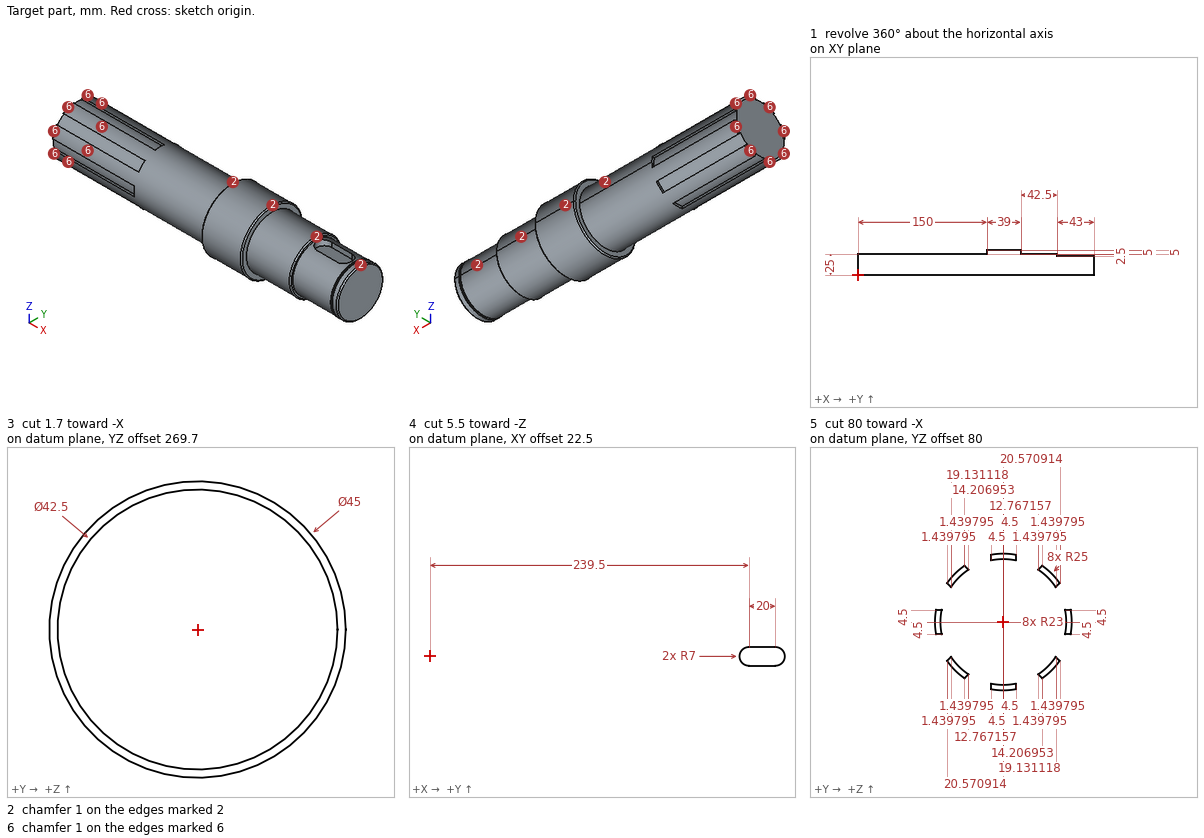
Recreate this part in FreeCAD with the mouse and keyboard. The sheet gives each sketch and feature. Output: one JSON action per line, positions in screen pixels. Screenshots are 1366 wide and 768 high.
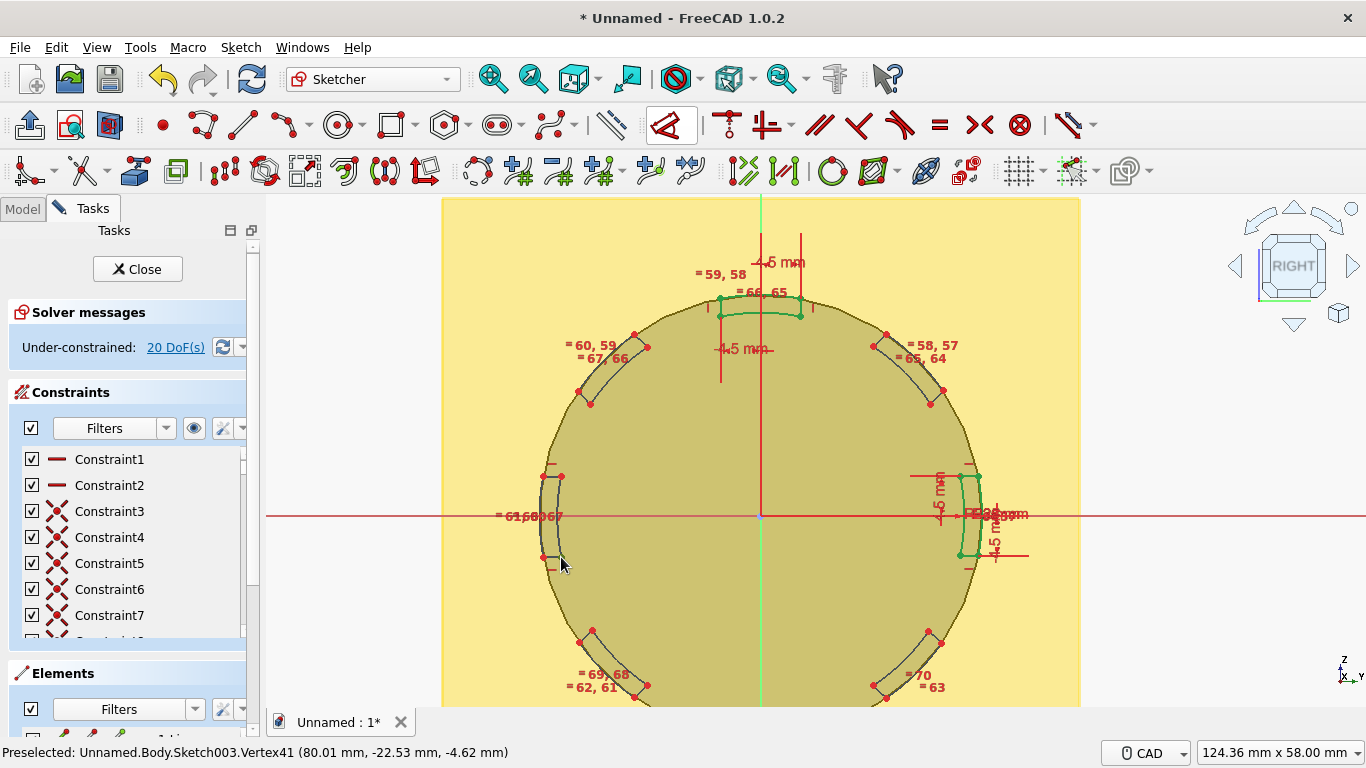
{"action": "left_click", "coordinate": [692, 126]}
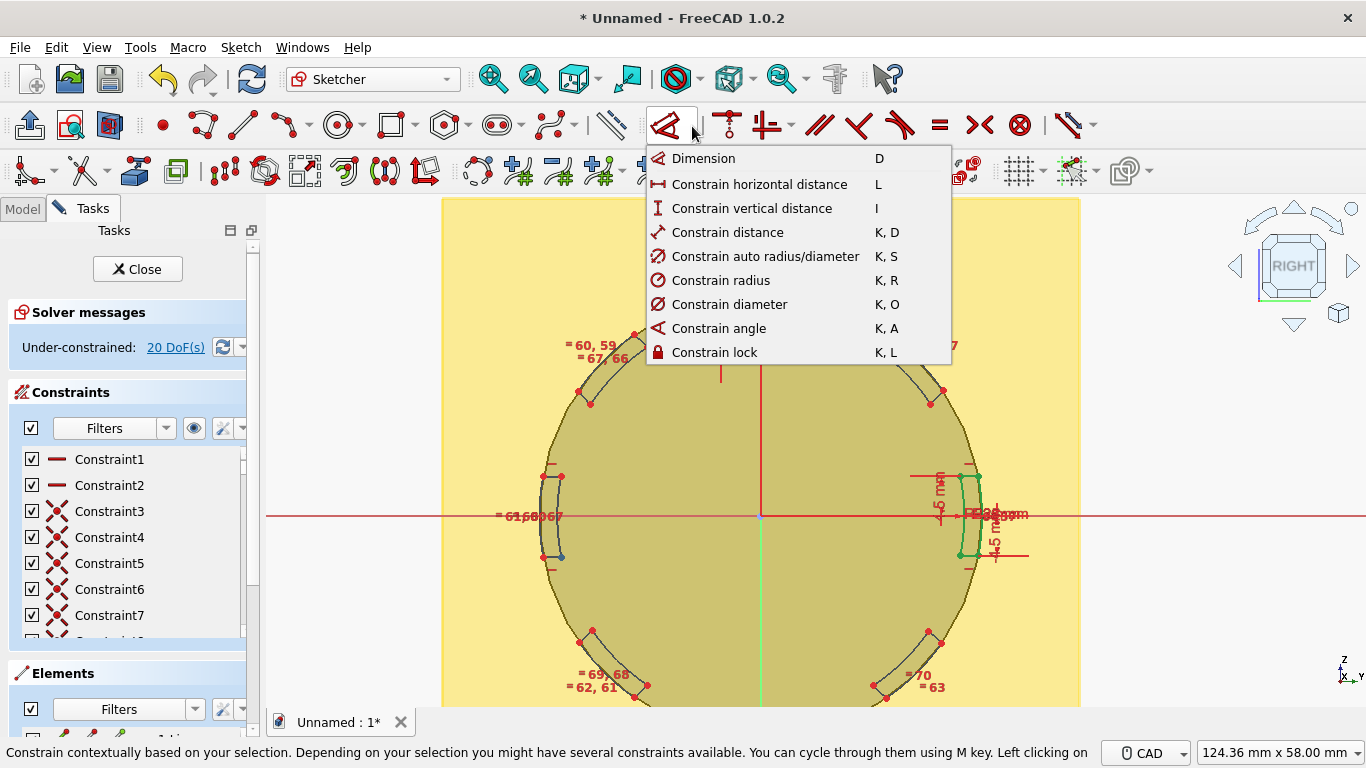
{"action": "left_click", "coordinate": [799, 208]}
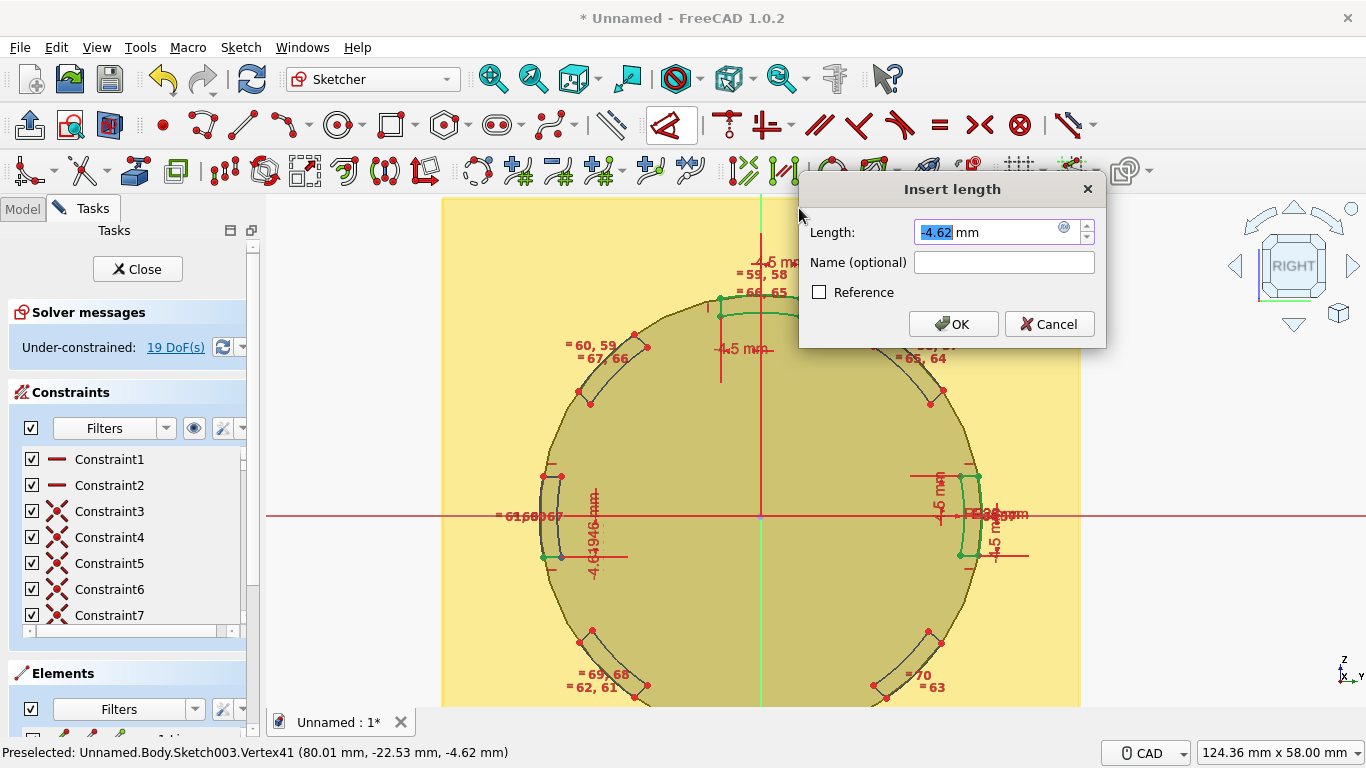
{"action": "type", "text": "-4.5"}
{"action": "key", "text": "Return"}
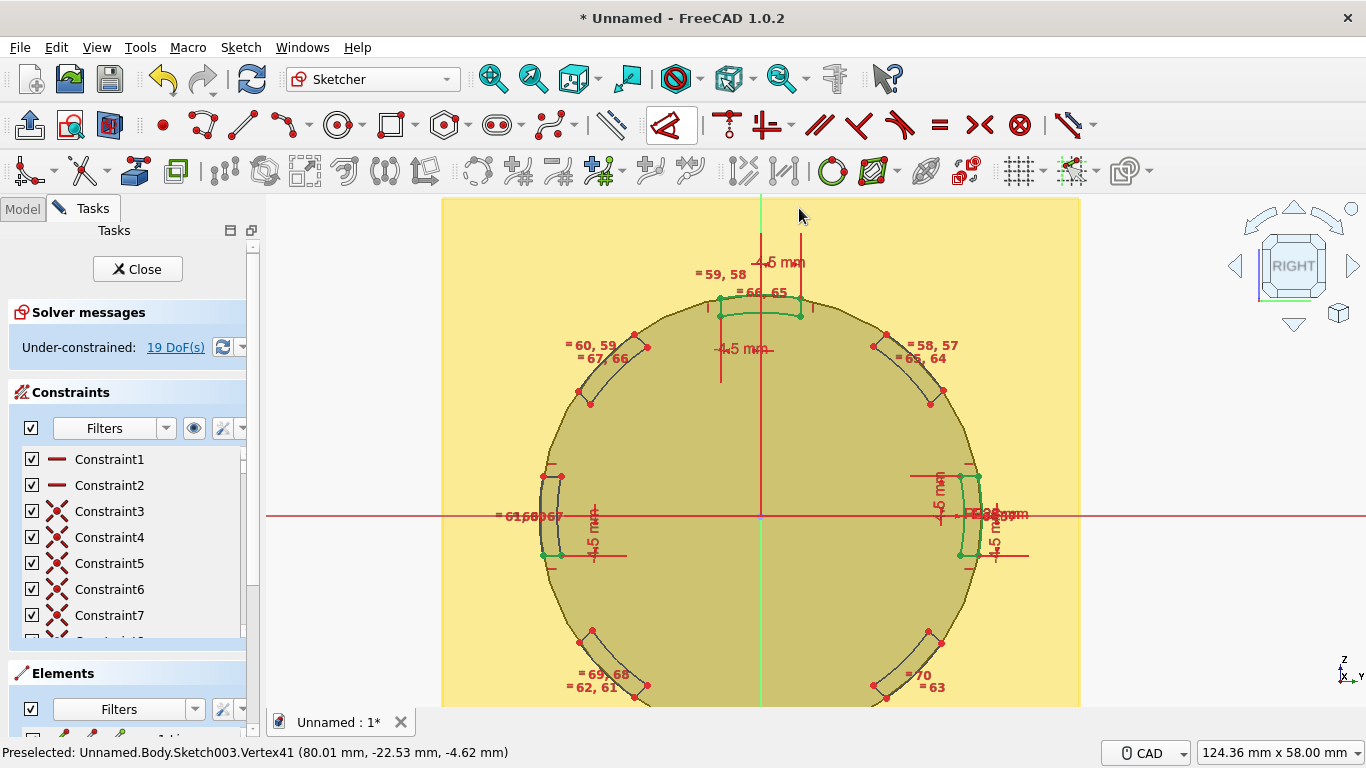
{"action": "left_click", "coordinate": [543, 477]}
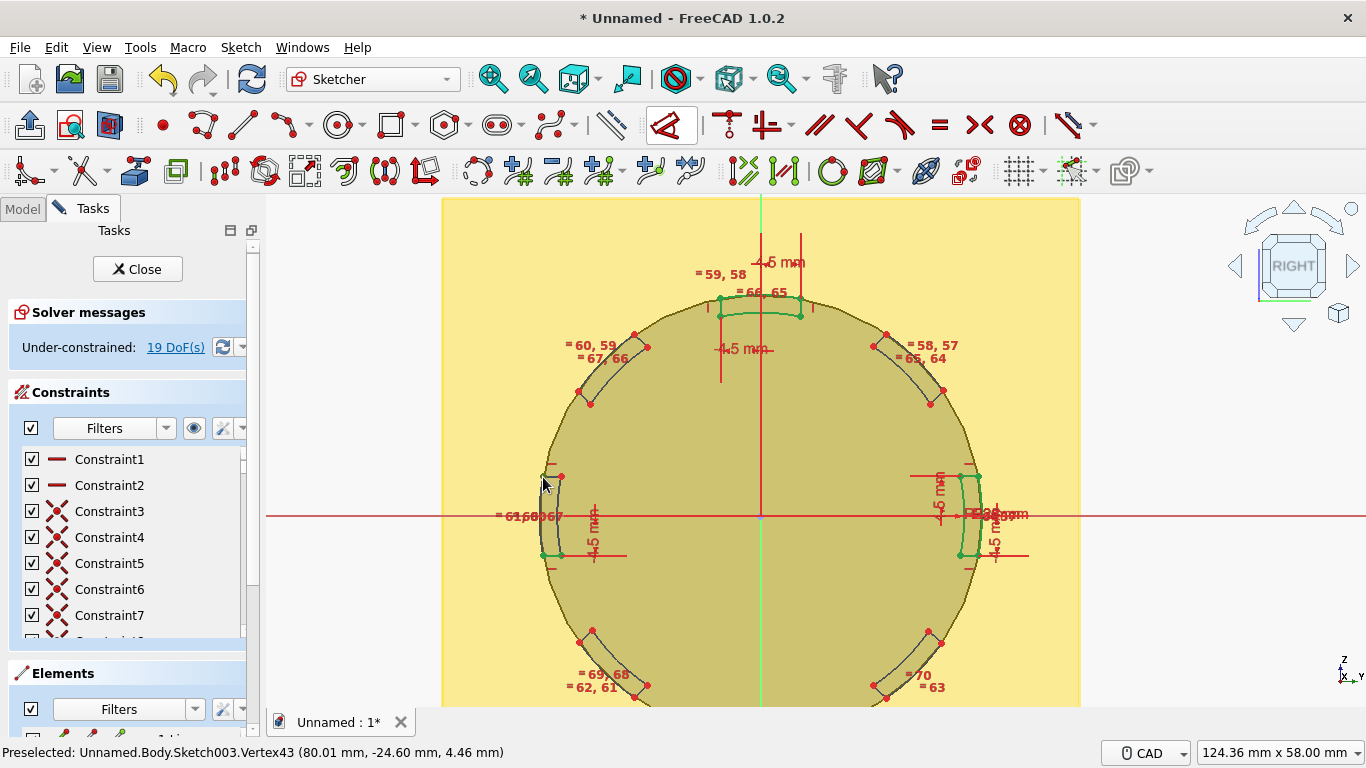
{"action": "key", "text": "i"}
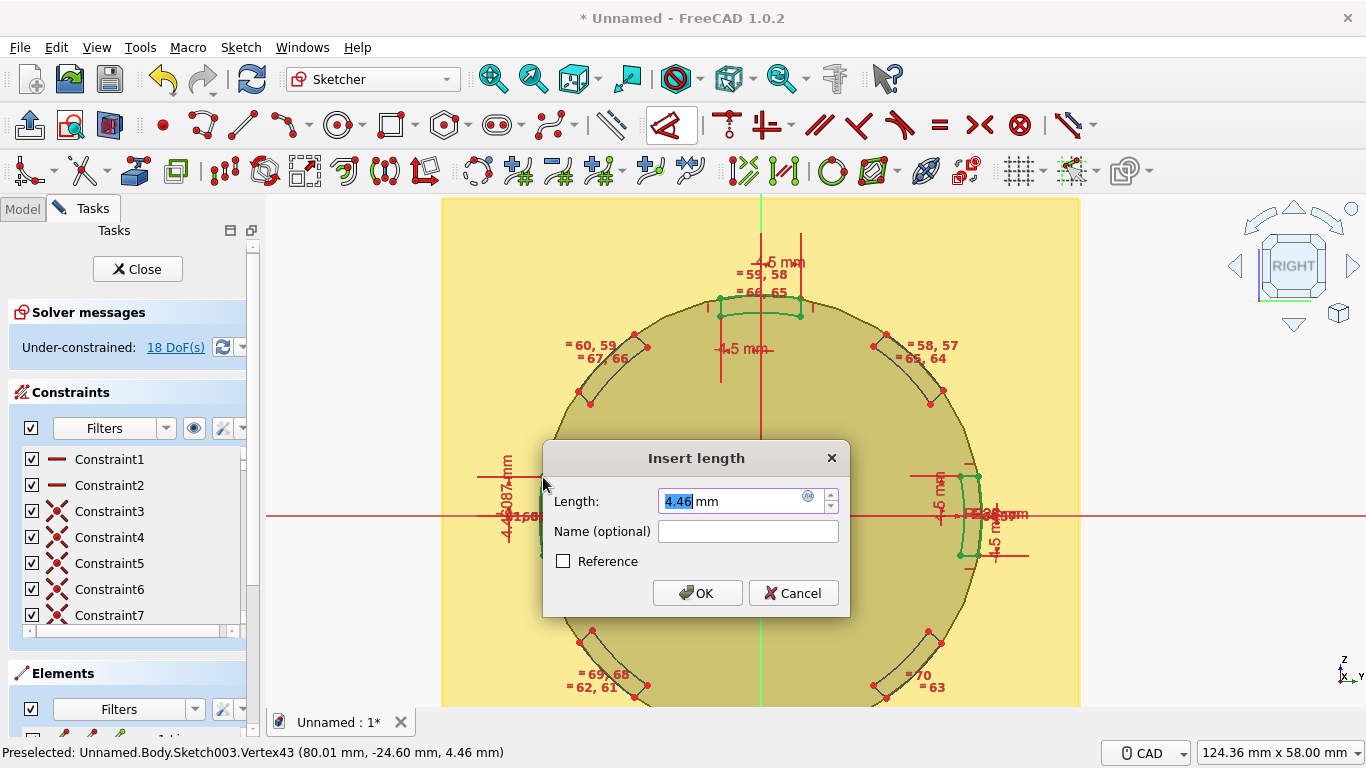
{"action": "type", "text": "4.5"}
{"action": "key", "text": "Return"}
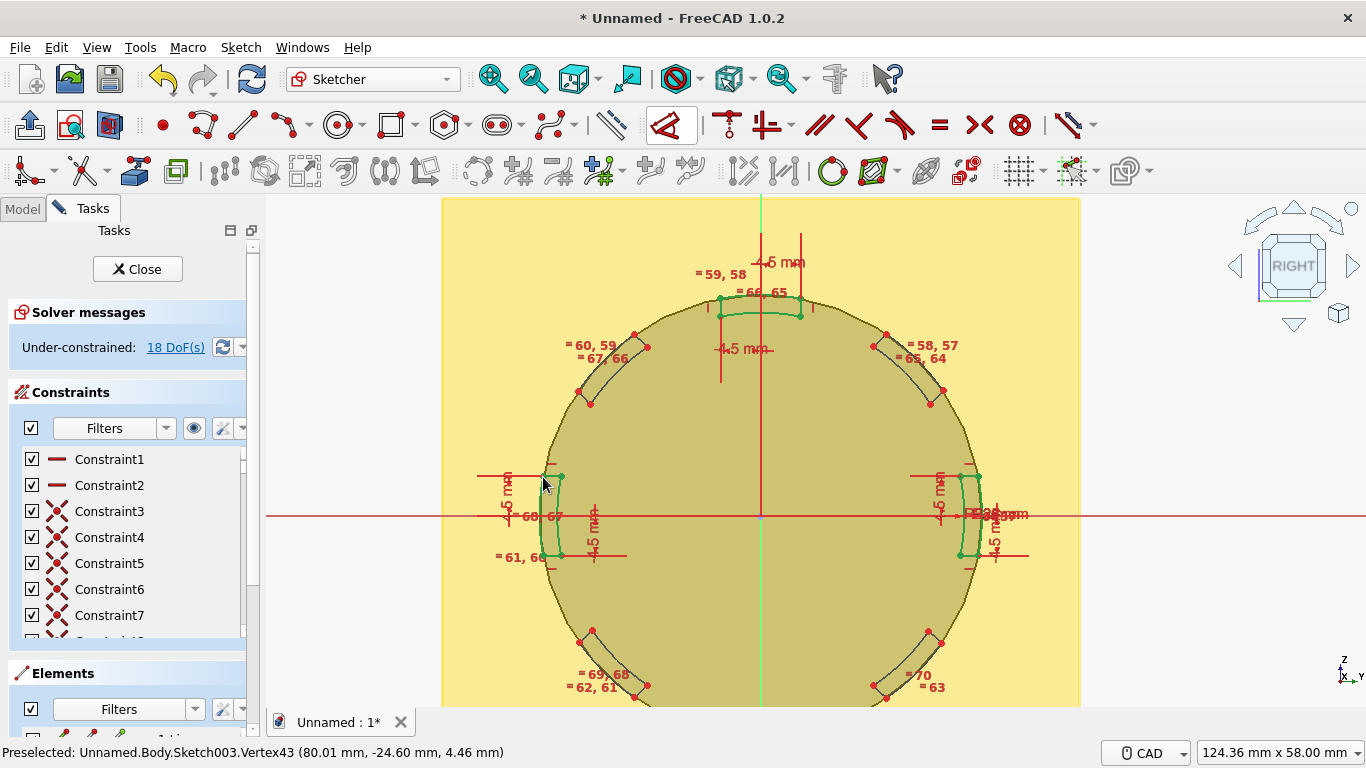
{"action": "scroll", "coordinate": [721, 317], "scroll_direction": "down", "scroll_amount": 2}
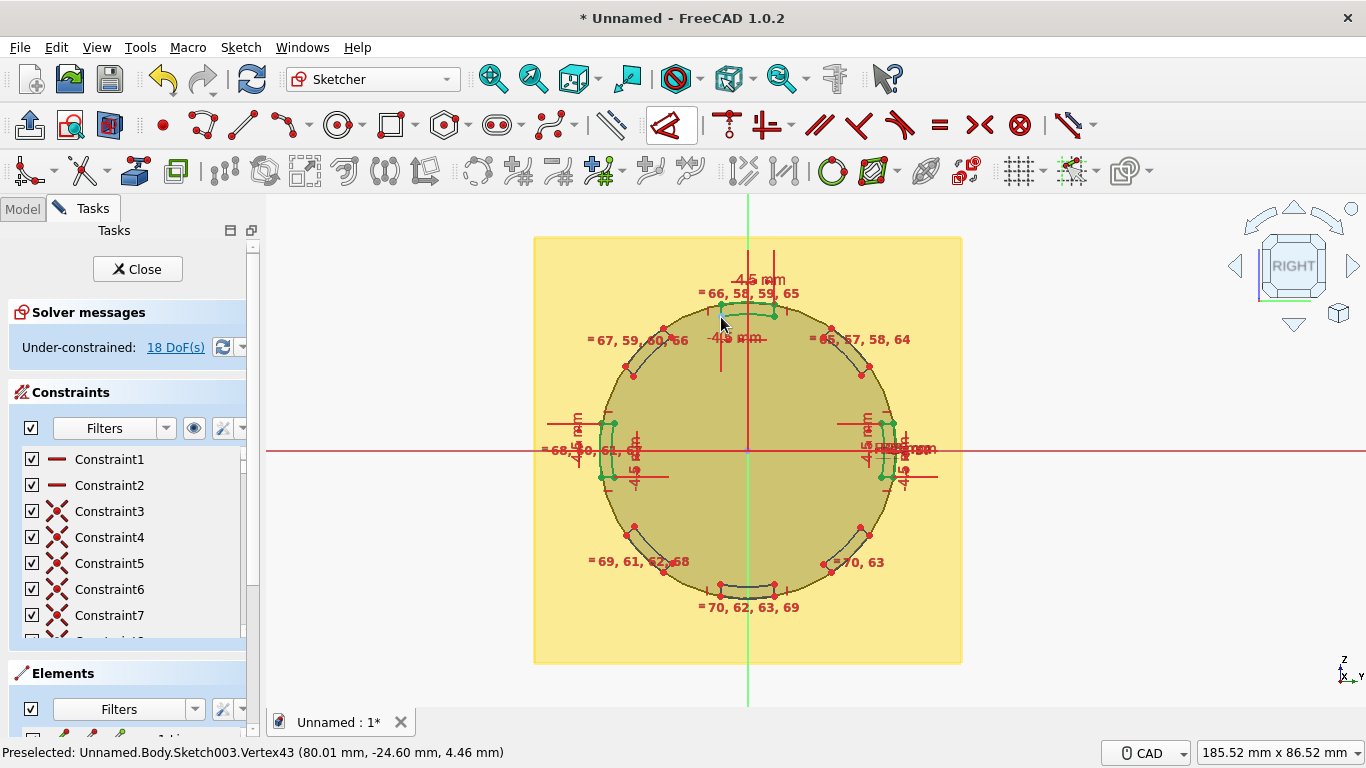
{"action": "scroll", "coordinate": [774, 584], "scroll_direction": "up", "scroll_amount": 2}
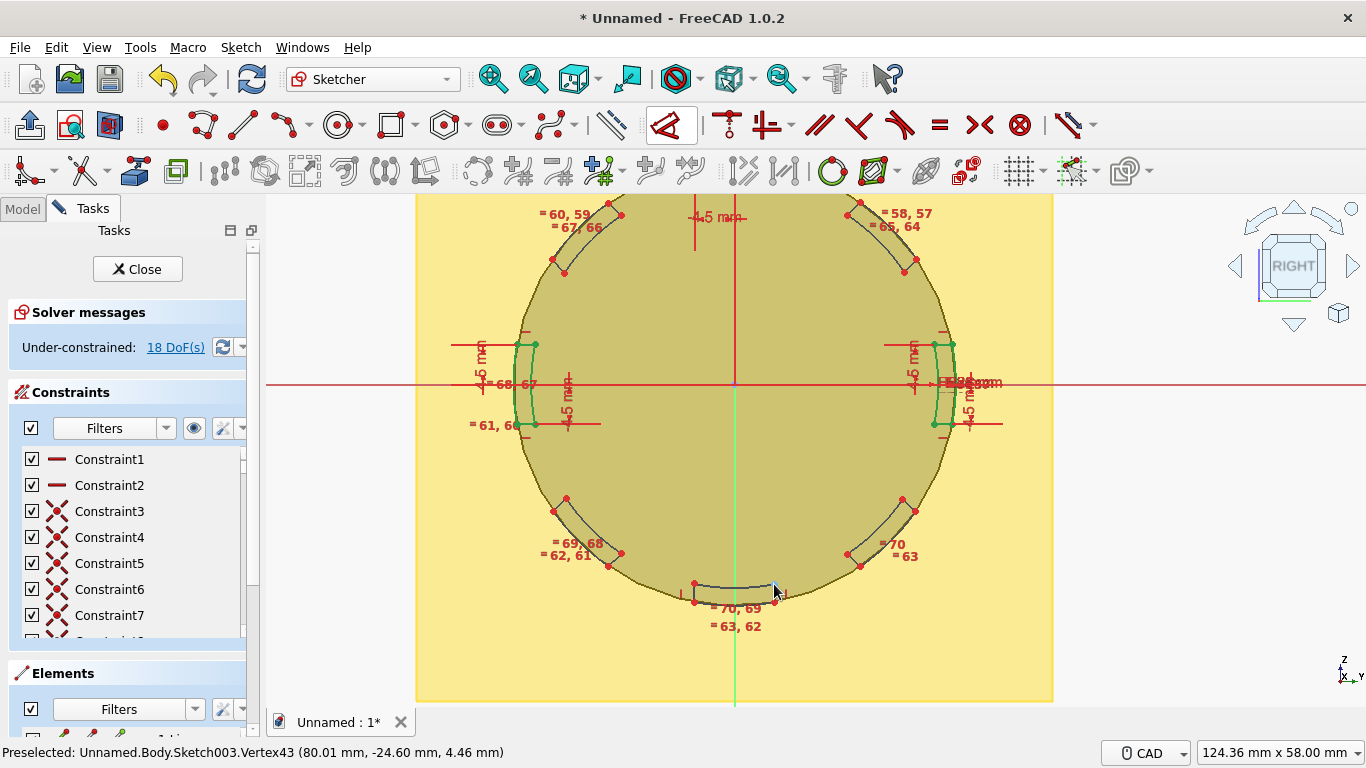
{"action": "left_click", "coordinate": [774, 584]}